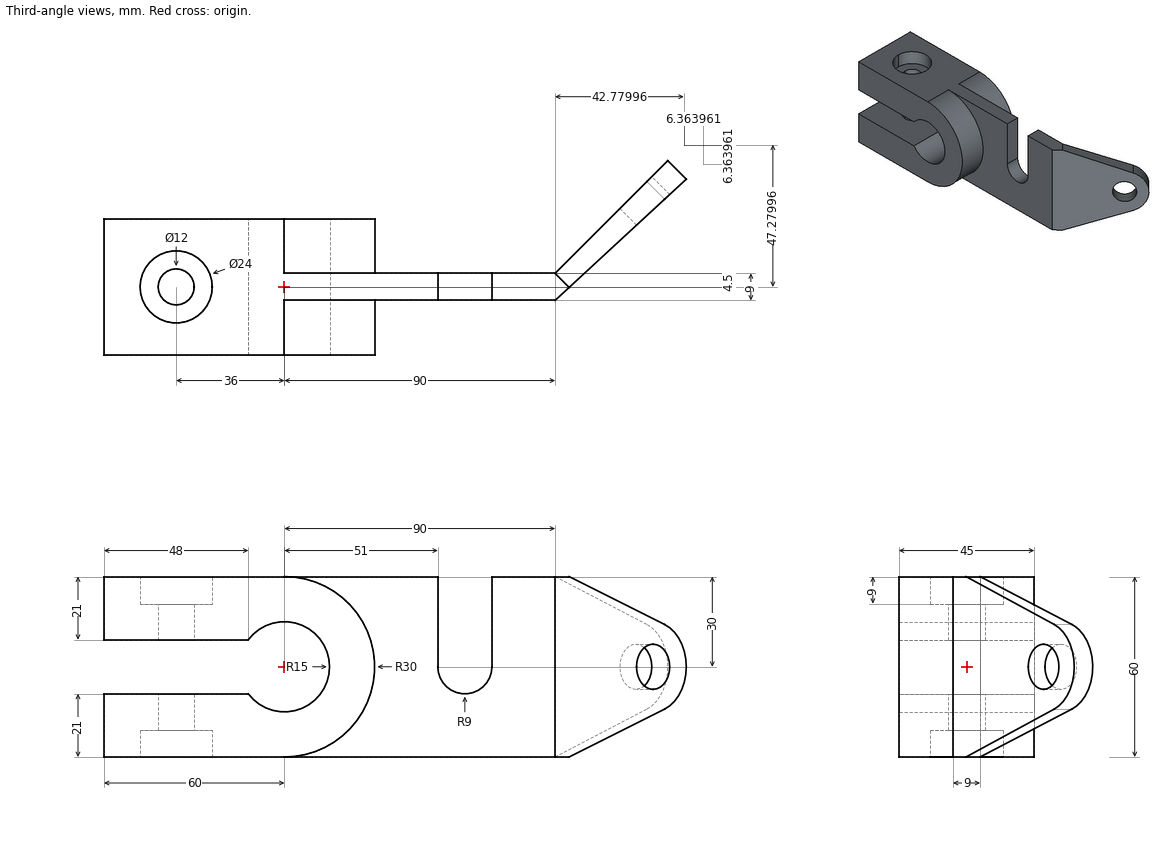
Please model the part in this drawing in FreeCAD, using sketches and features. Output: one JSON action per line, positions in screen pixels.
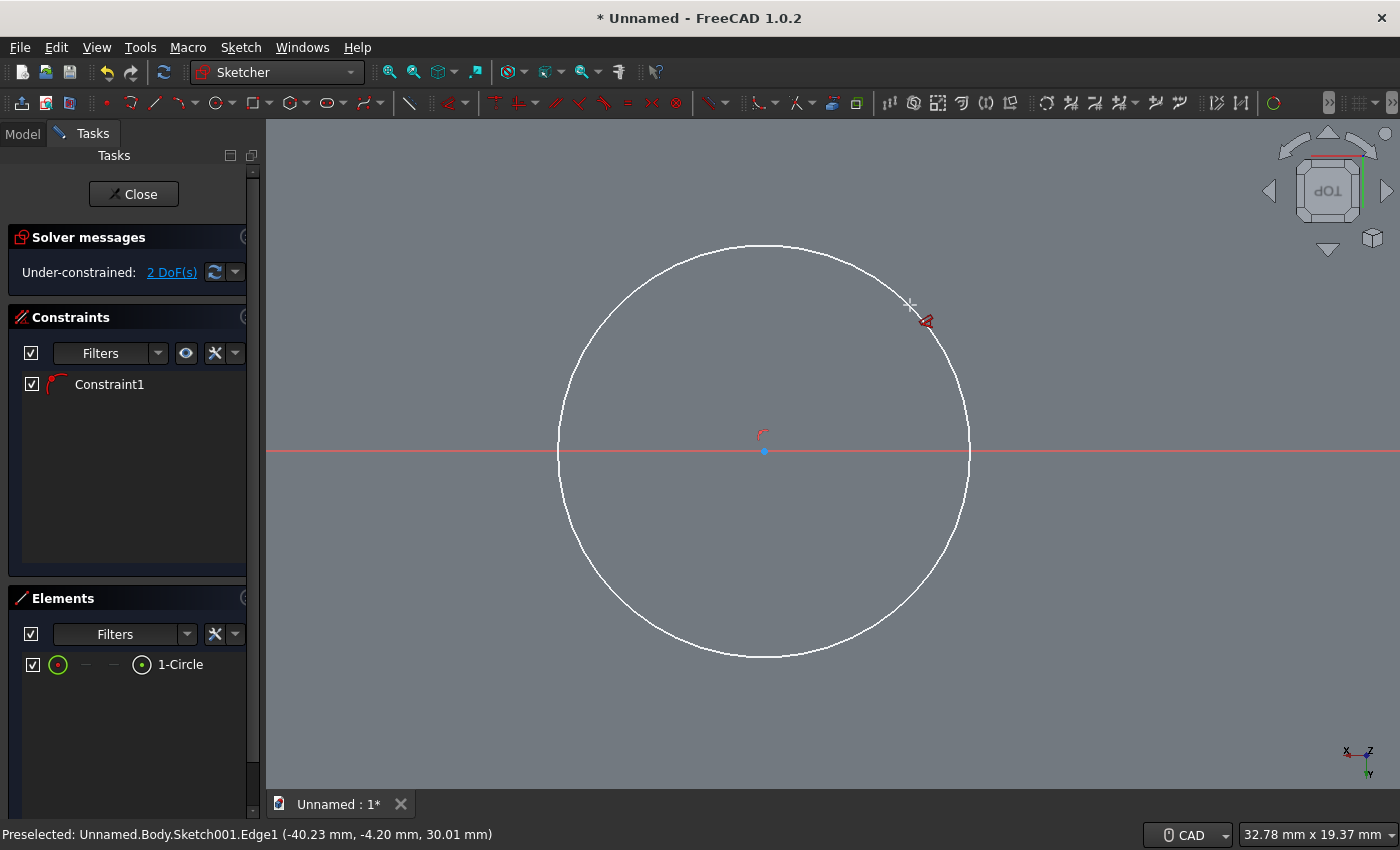
{"action": "left_click", "coordinate": [909, 305]}
{"action": "left_click", "coordinate": [932, 282]}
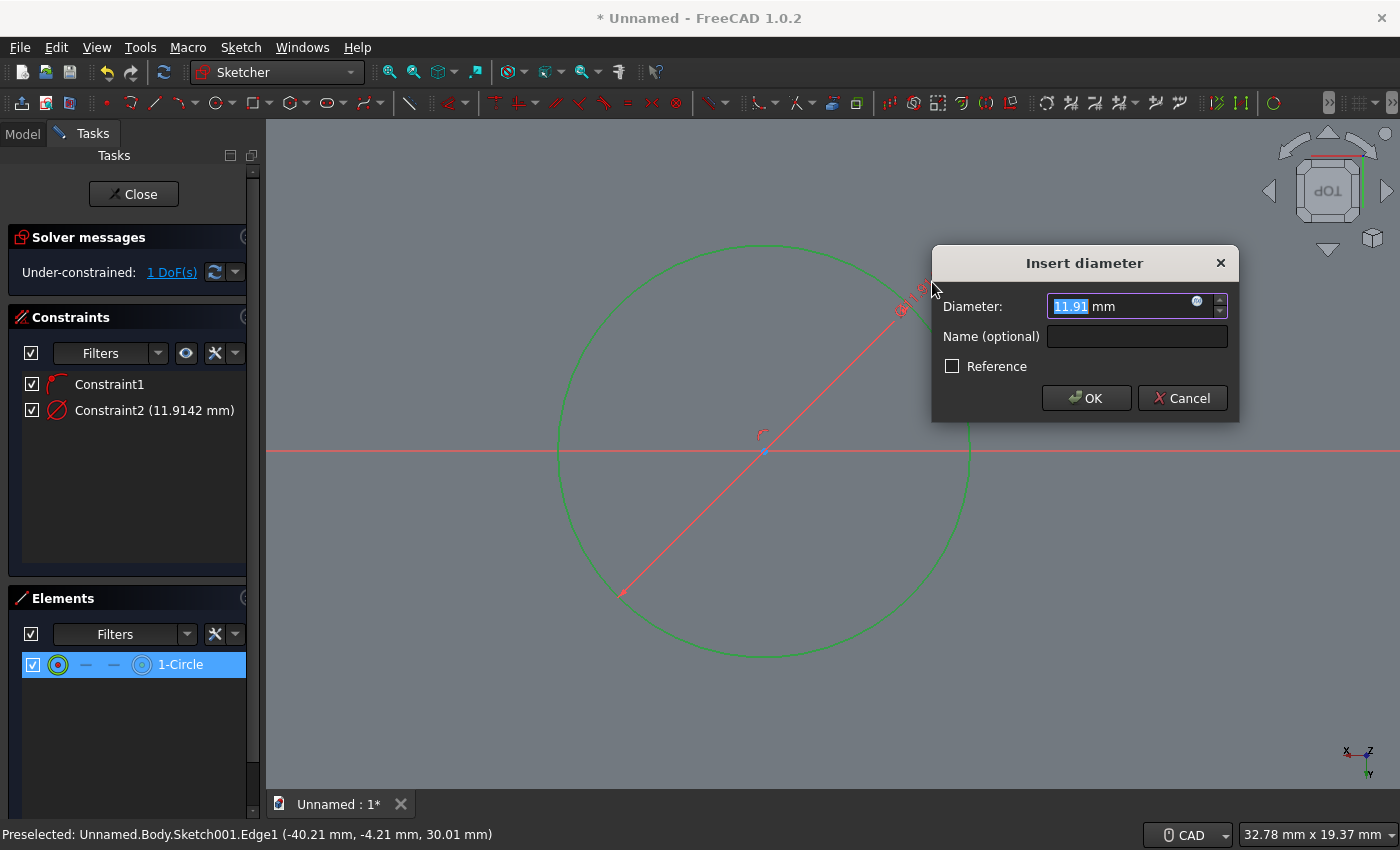
{"action": "type", "text": "12"}
{"action": "key", "text": "Return"}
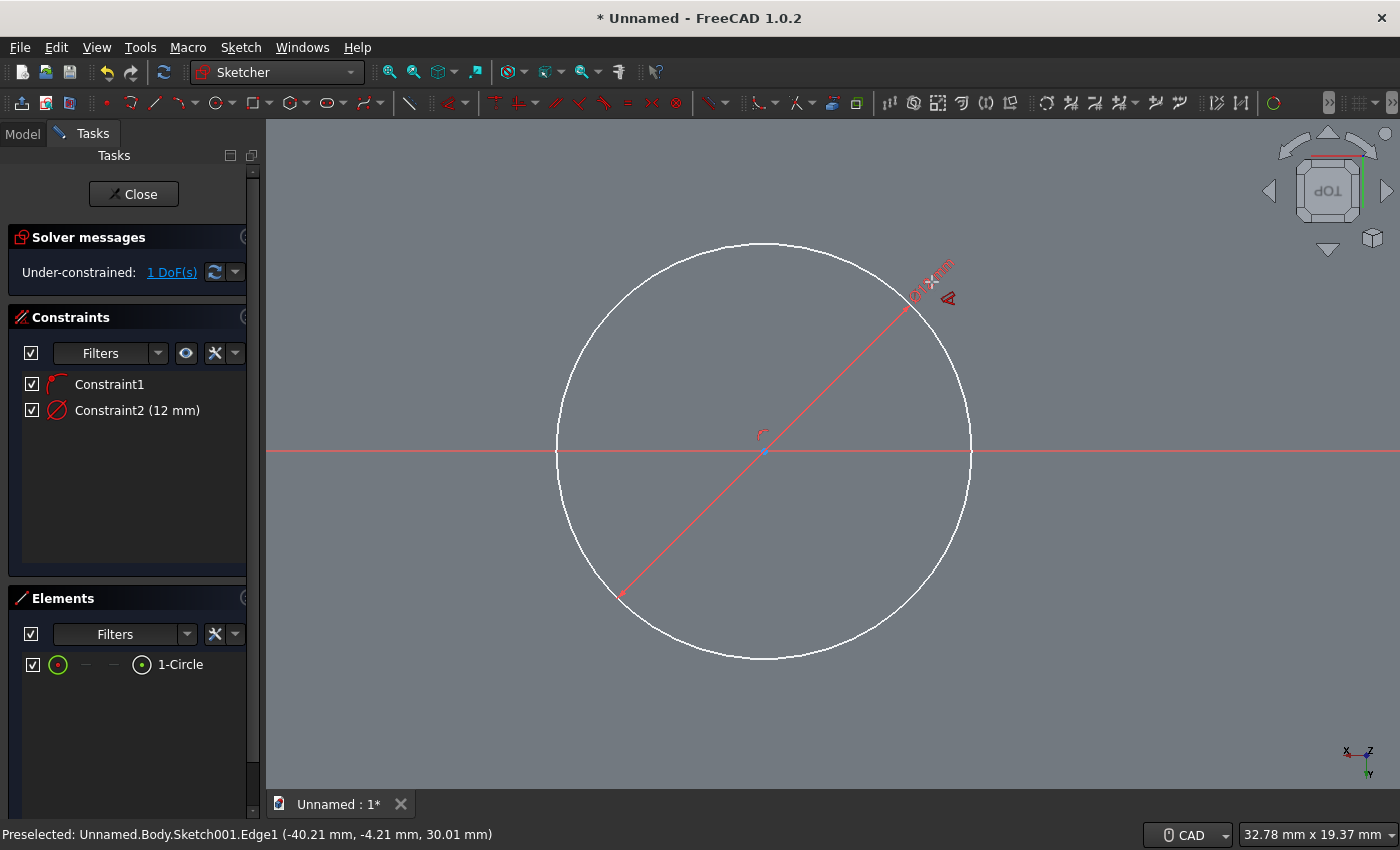
{"action": "left_click", "coordinate": [764, 451]}
{"action": "left_click", "coordinate": [529, 485]}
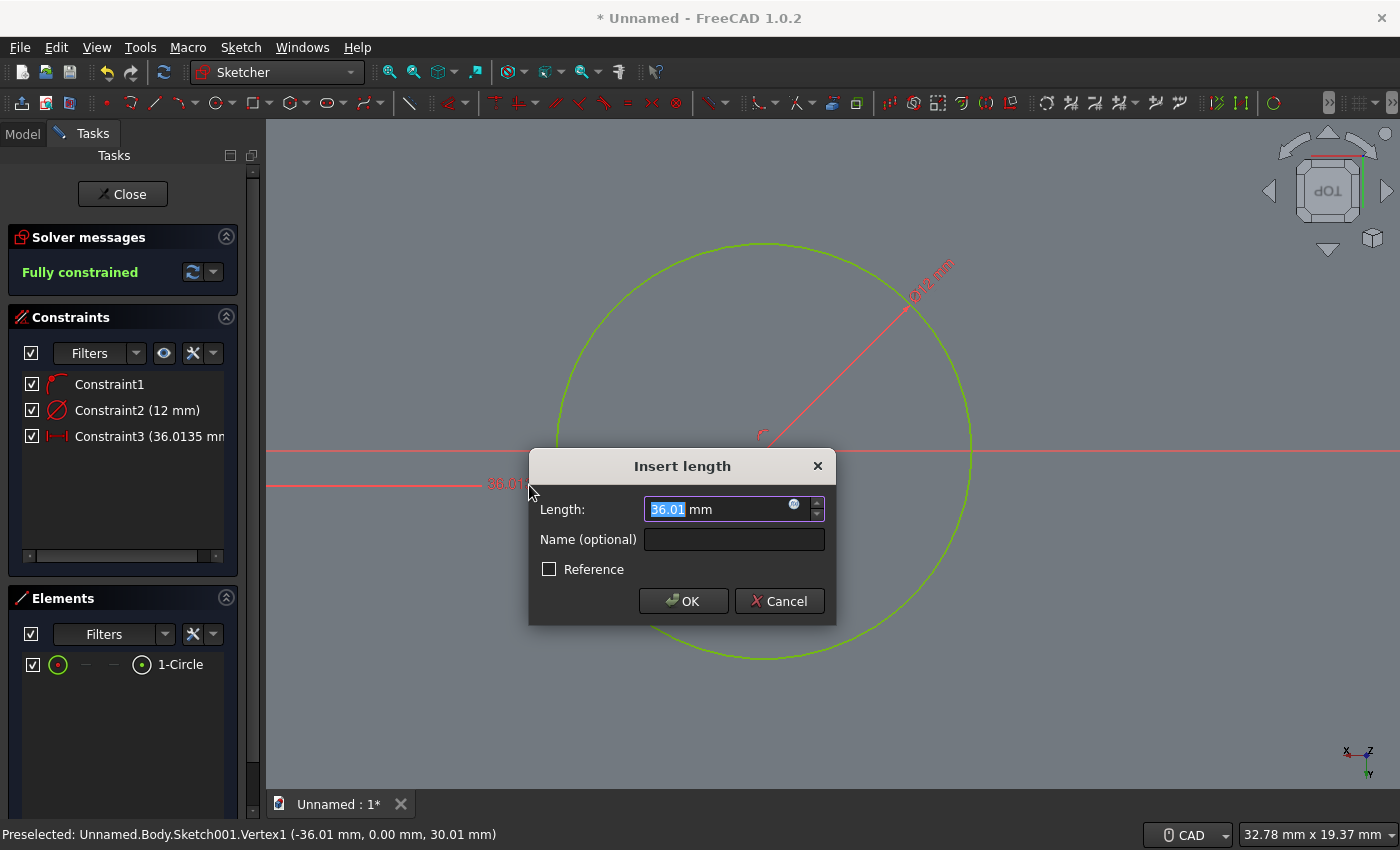
{"action": "type", "text": "36"}
{"action": "key", "text": "Return"}
{"action": "key", "text": "Escape"}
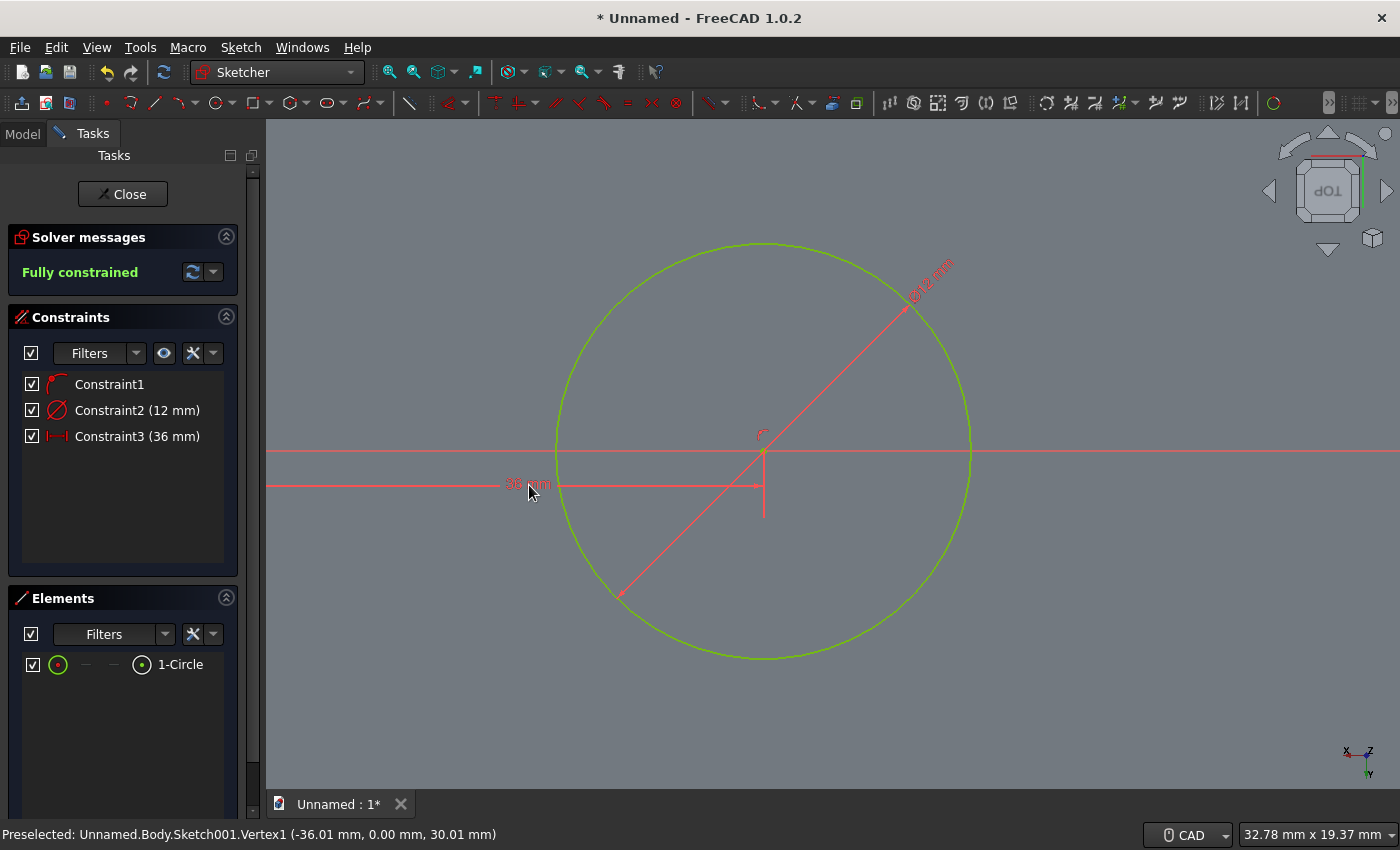
{"action": "left_click", "coordinate": [123, 194]}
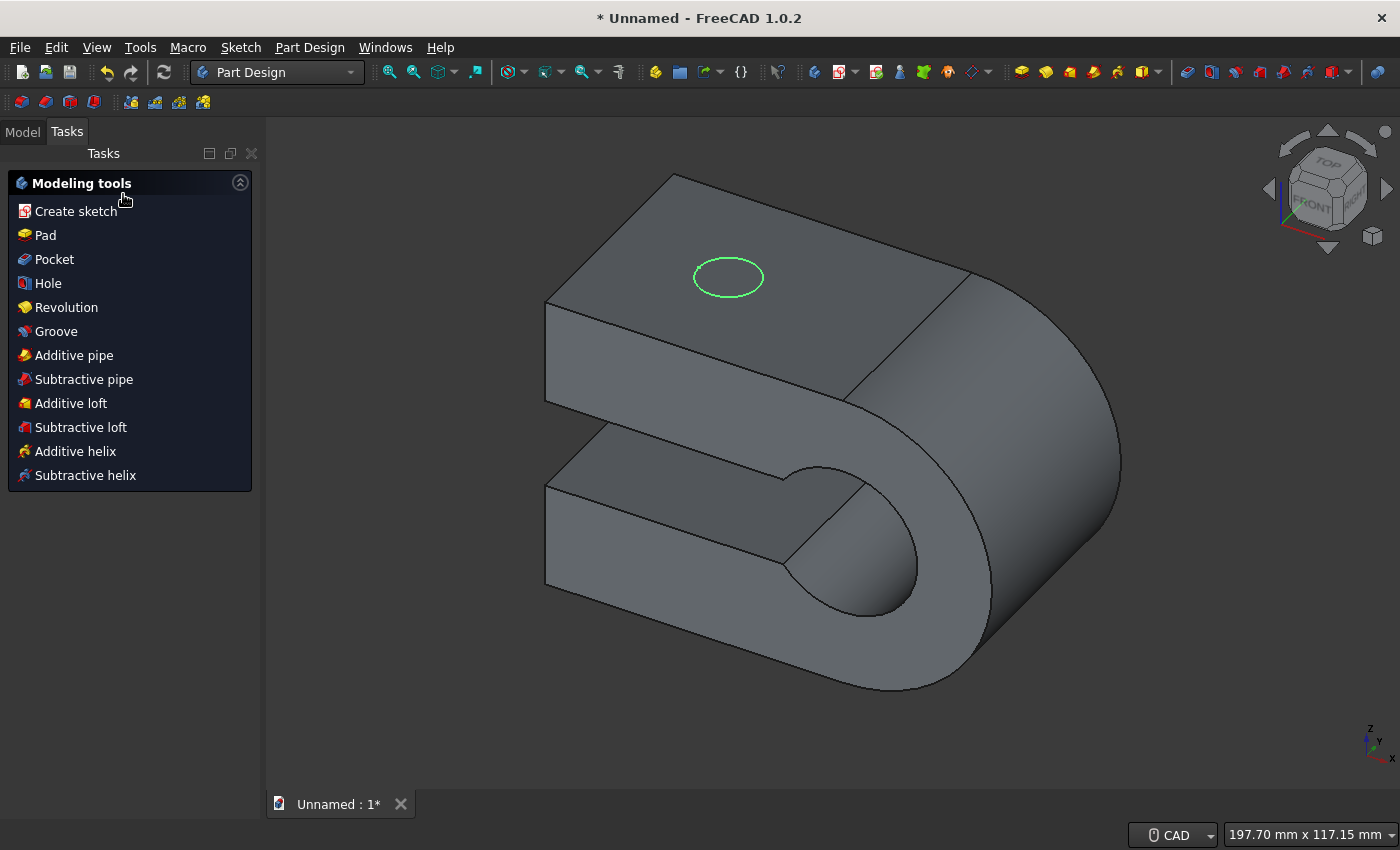
{"action": "left_click", "coordinate": [1188, 72]}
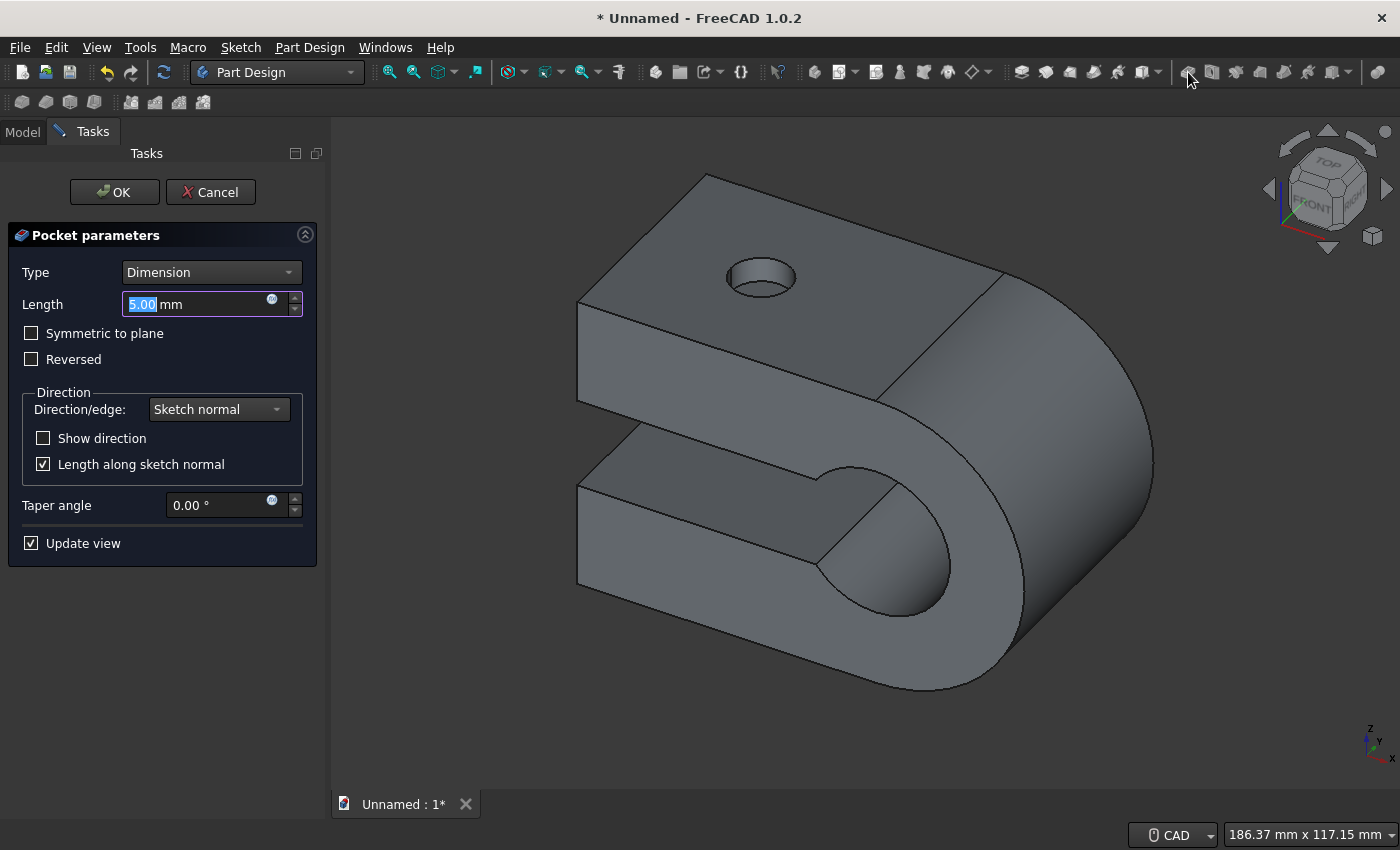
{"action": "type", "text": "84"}
{"action": "key", "text": "Tab"}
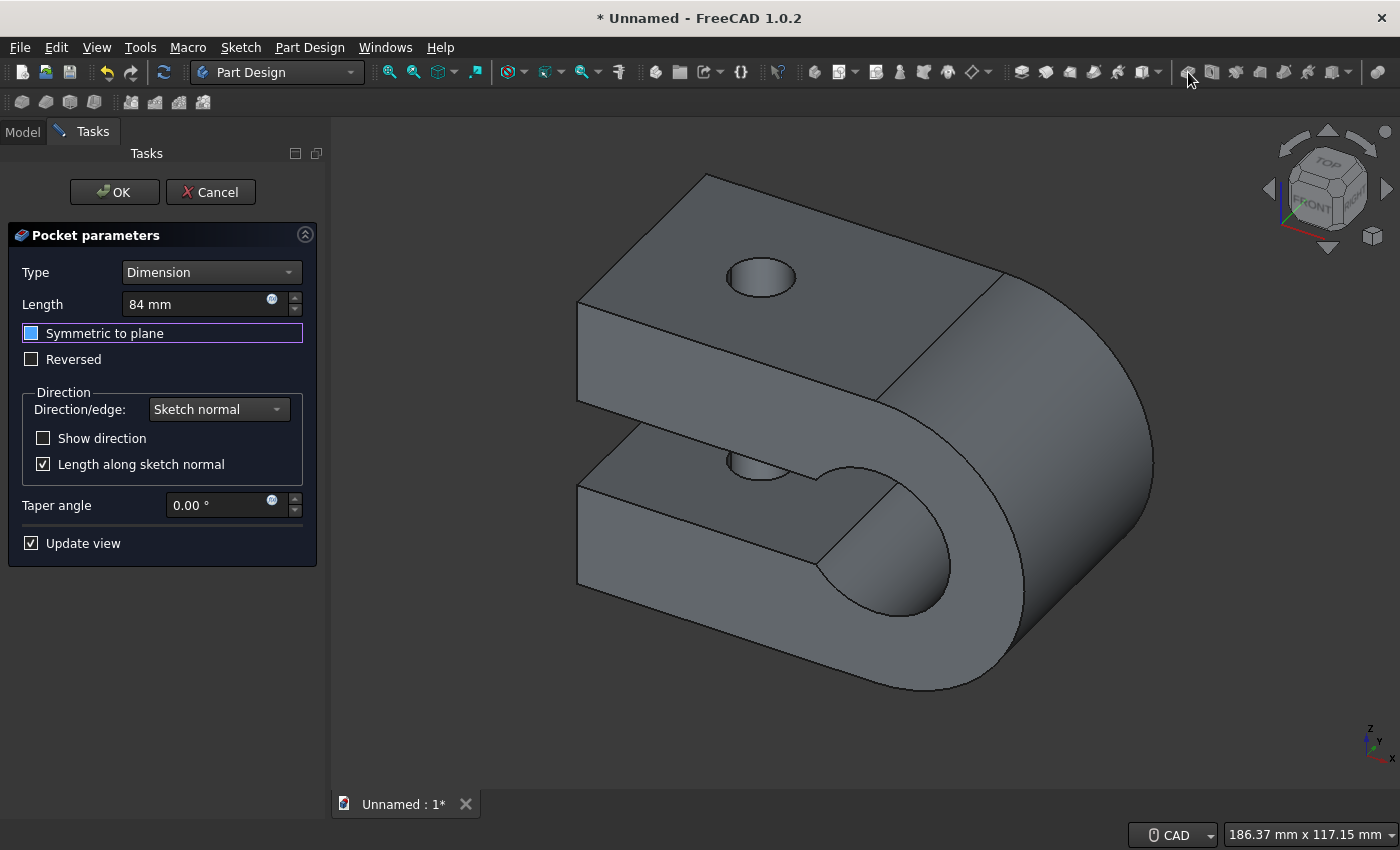
{"action": "left_click", "coordinate": [115, 192]}